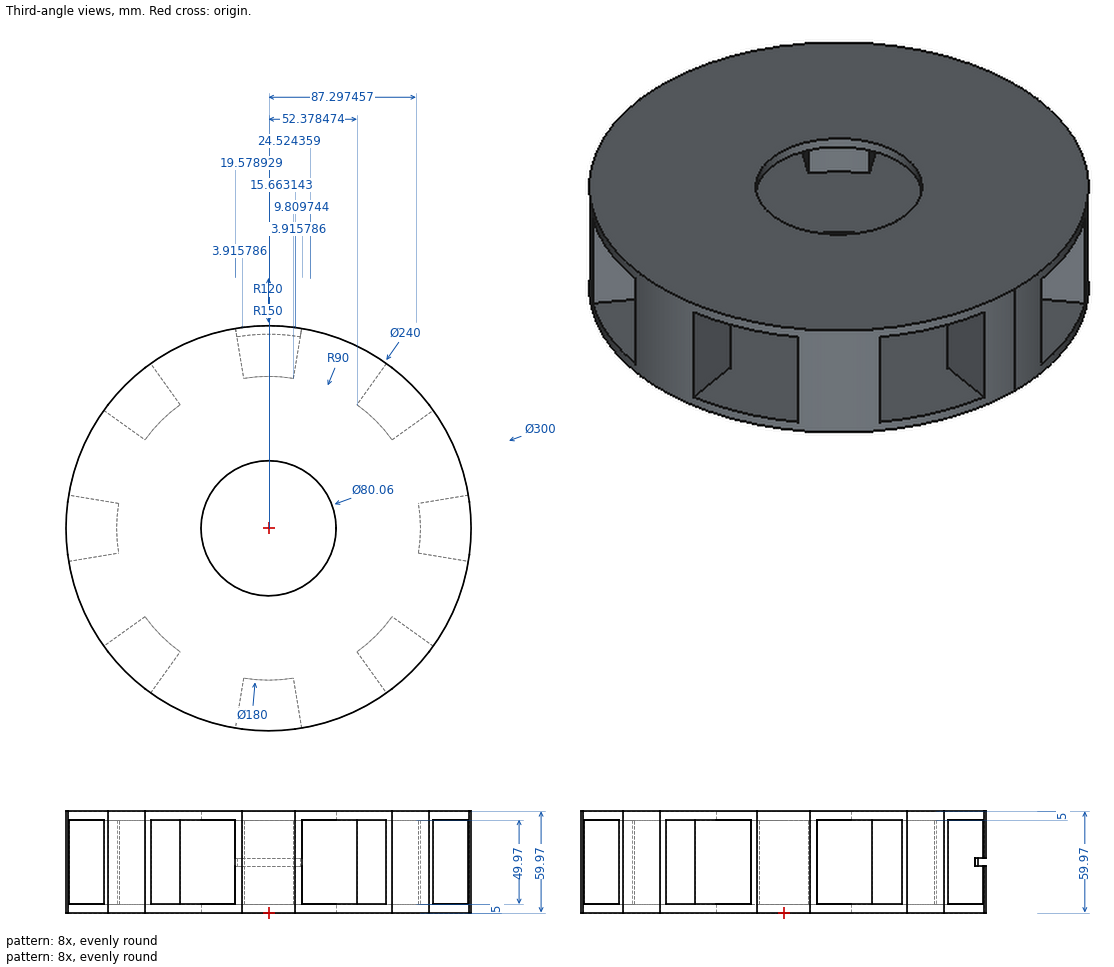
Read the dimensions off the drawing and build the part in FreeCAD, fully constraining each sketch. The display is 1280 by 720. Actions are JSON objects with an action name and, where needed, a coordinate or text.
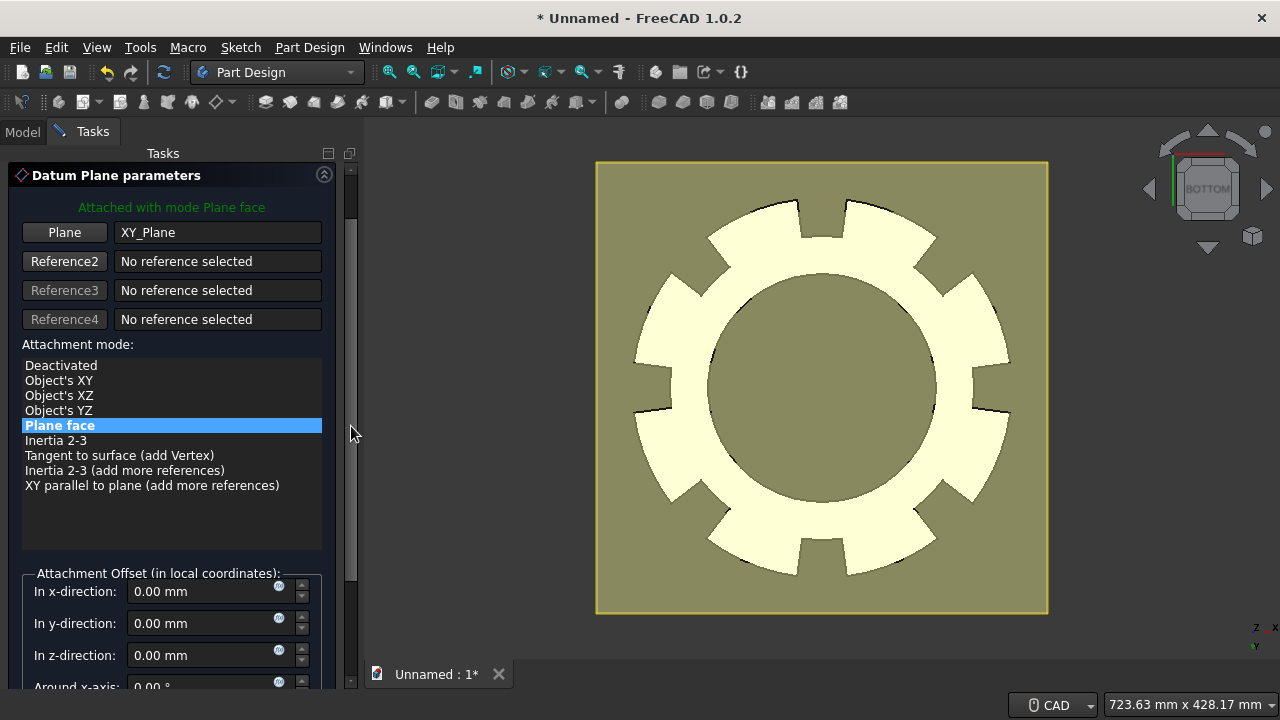
{"action": "triple_click", "coordinate": [210, 595]}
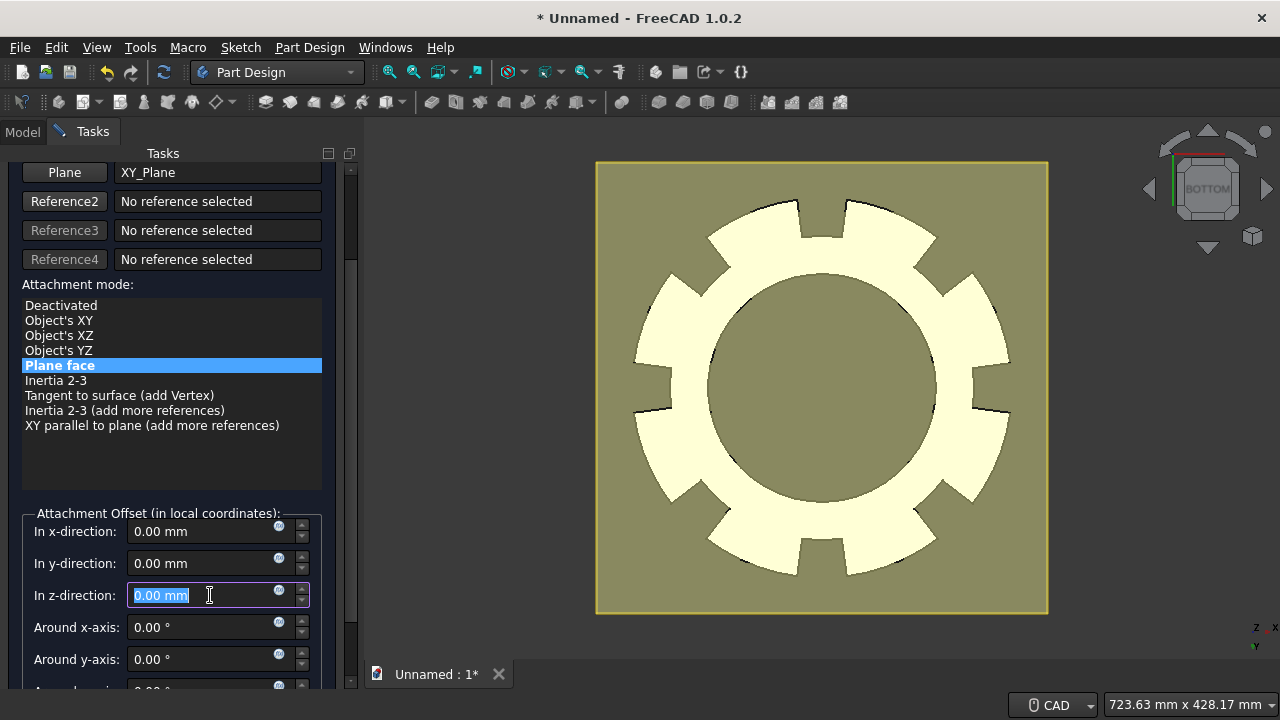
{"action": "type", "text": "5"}
{"action": "key", "text": "Tab"}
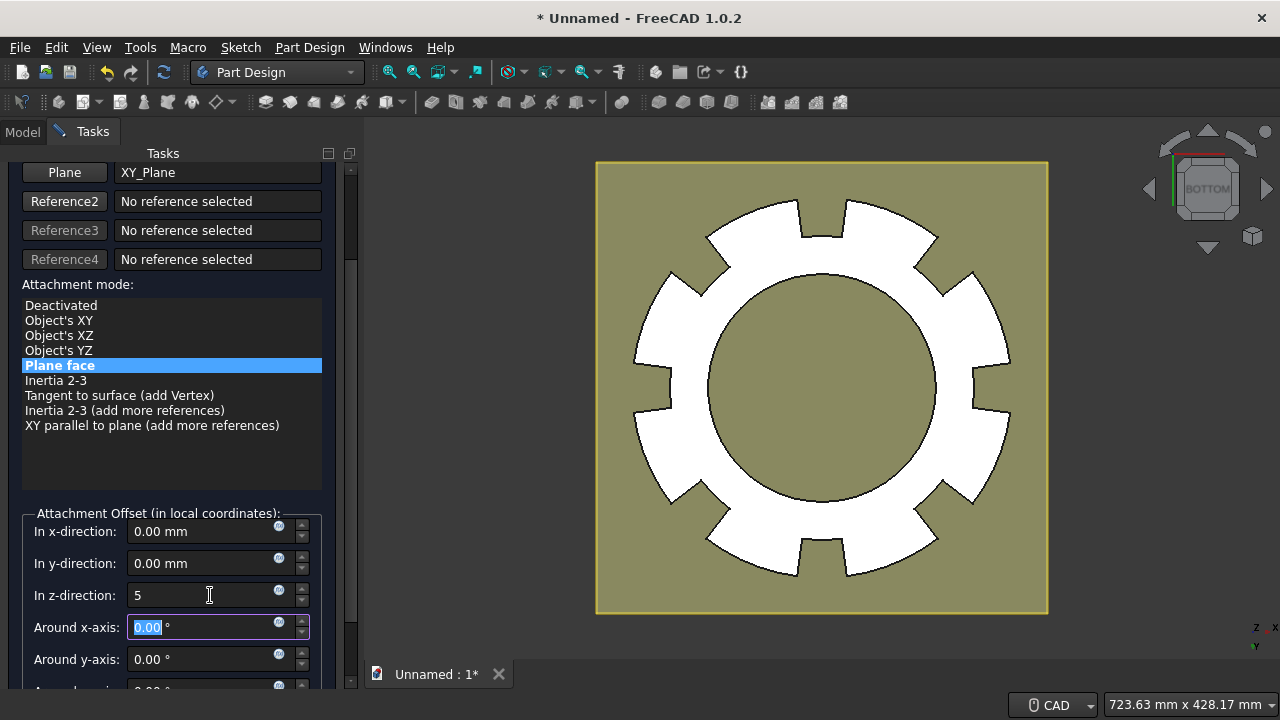
{"action": "scroll", "coordinate": [351, 426], "scroll_direction": "up", "scroll_amount": 3}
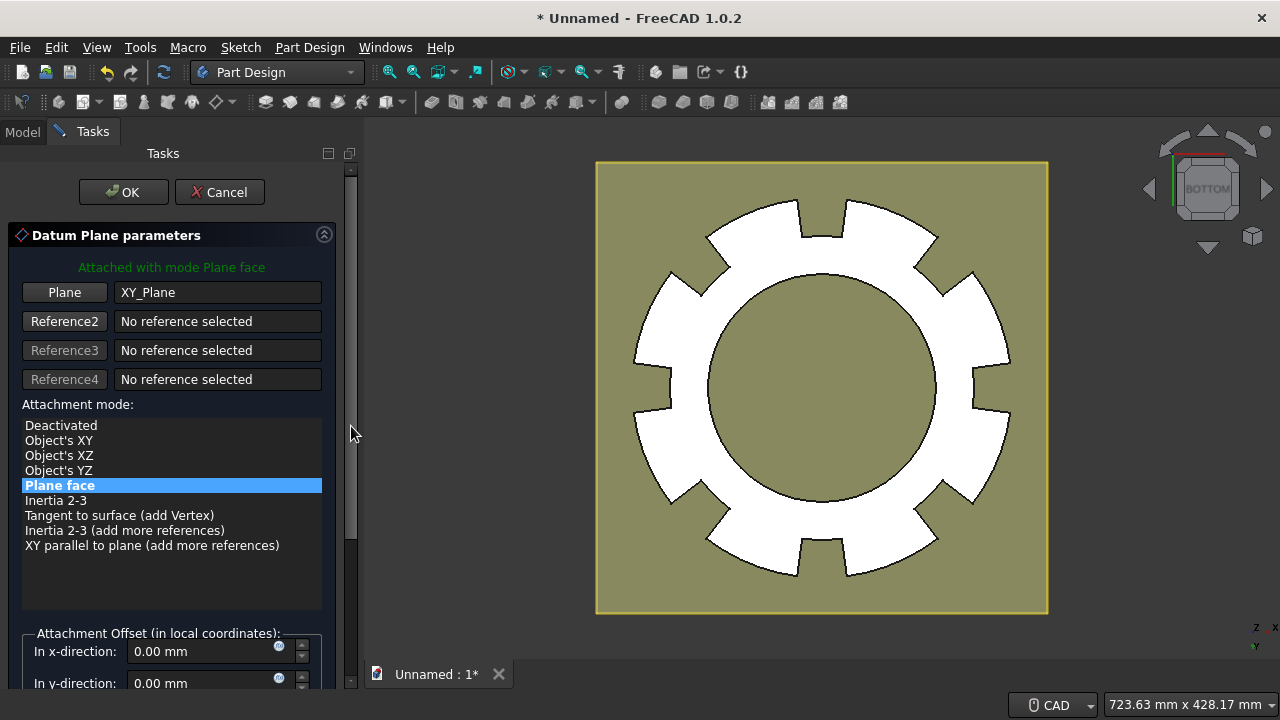
{"action": "left_click", "coordinate": [124, 192]}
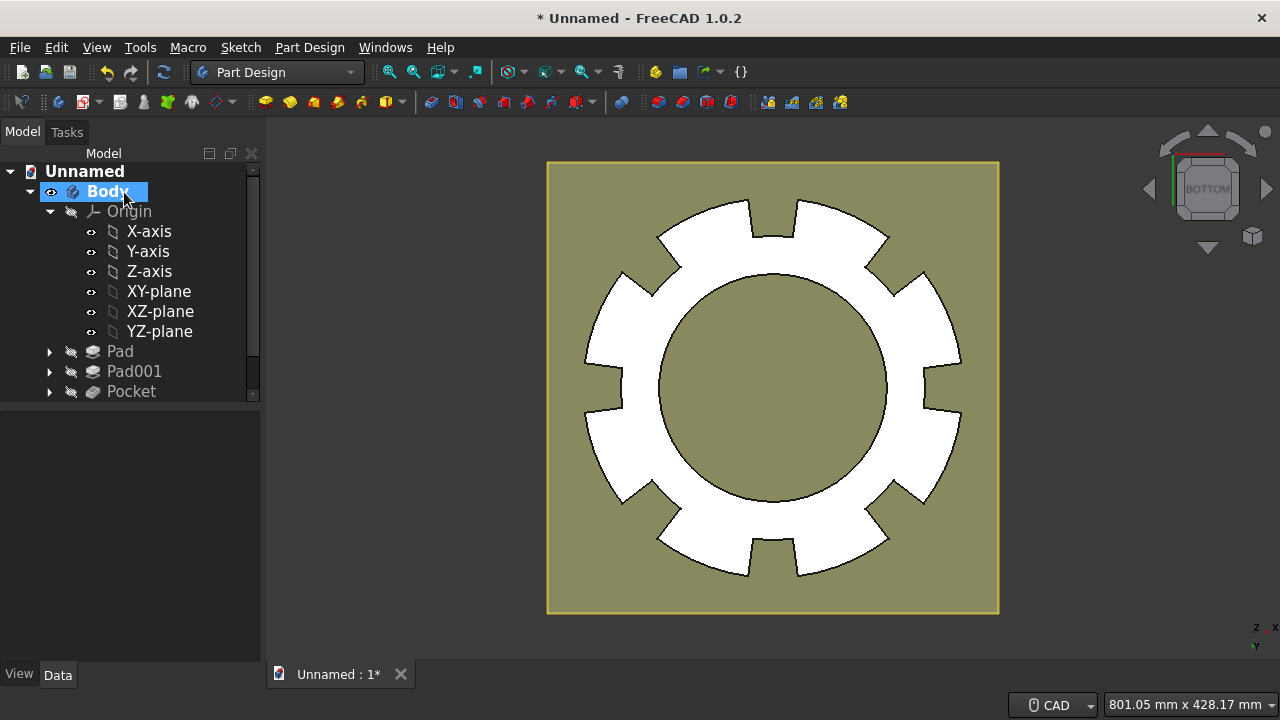
{"action": "scroll", "coordinate": [100, 287], "scroll_direction": "down", "scroll_amount": 3}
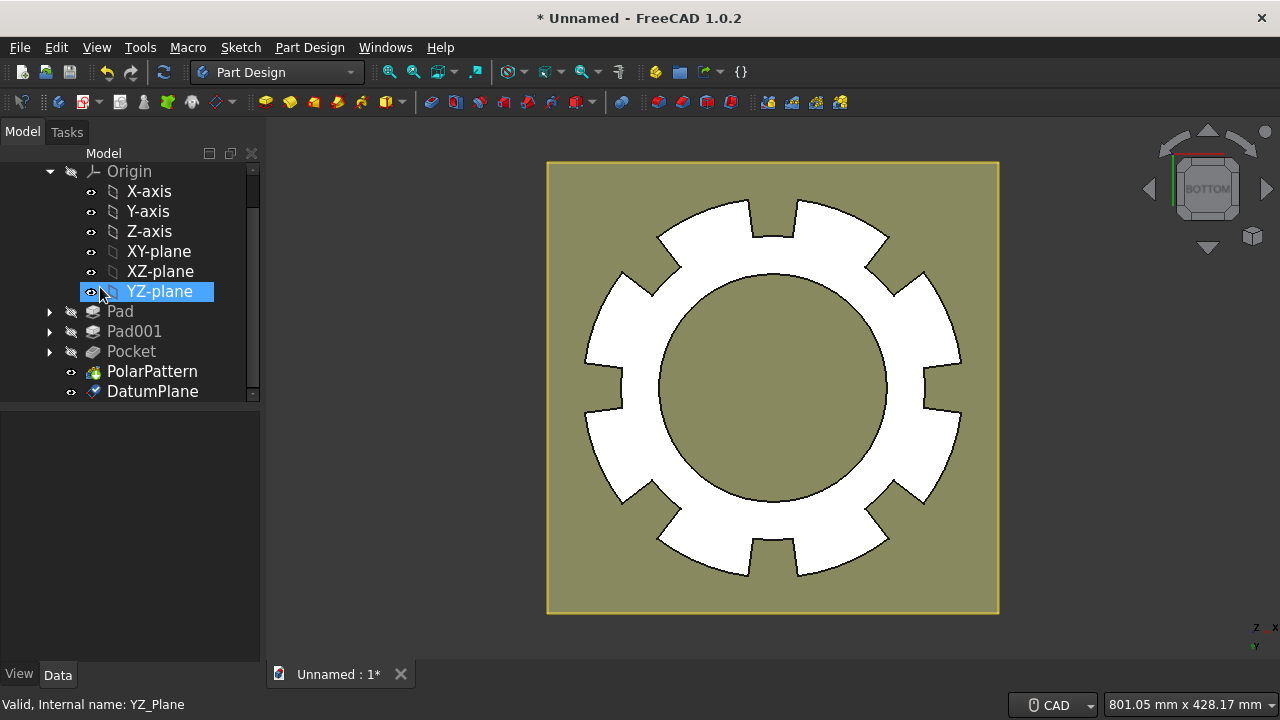
{"action": "left_click", "coordinate": [116, 392]}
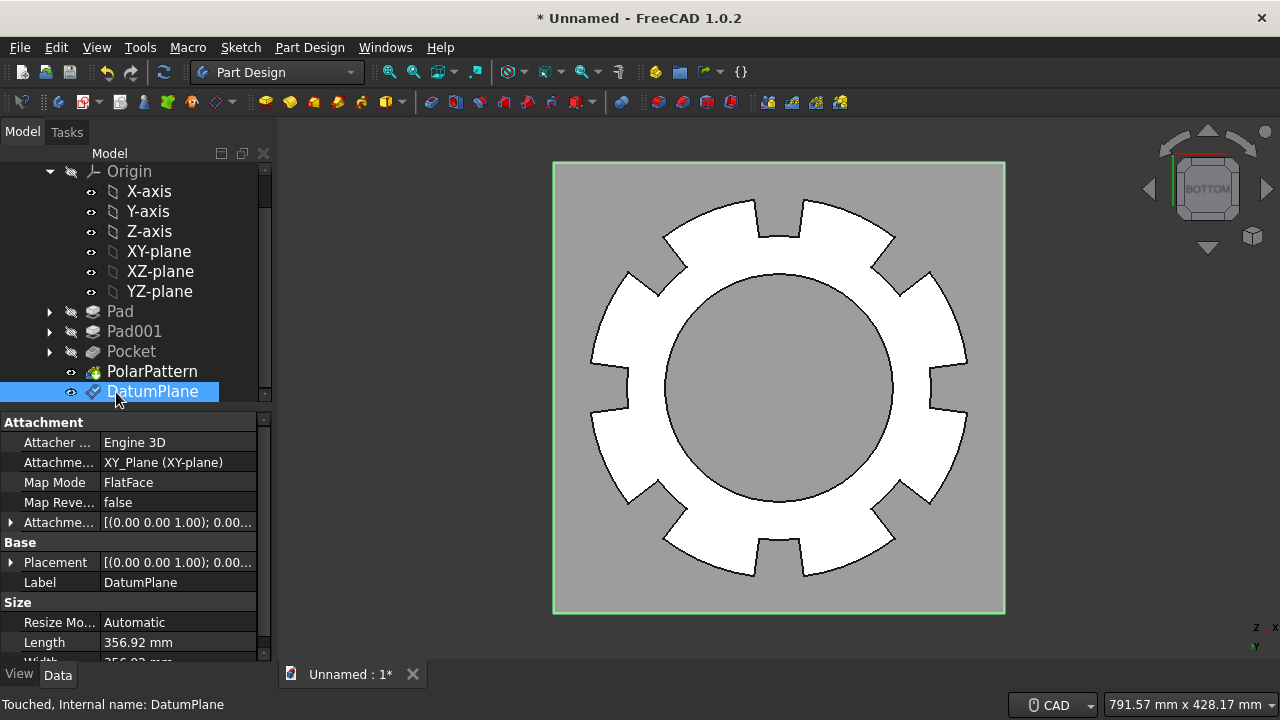
{"action": "left_click", "coordinate": [84, 102]}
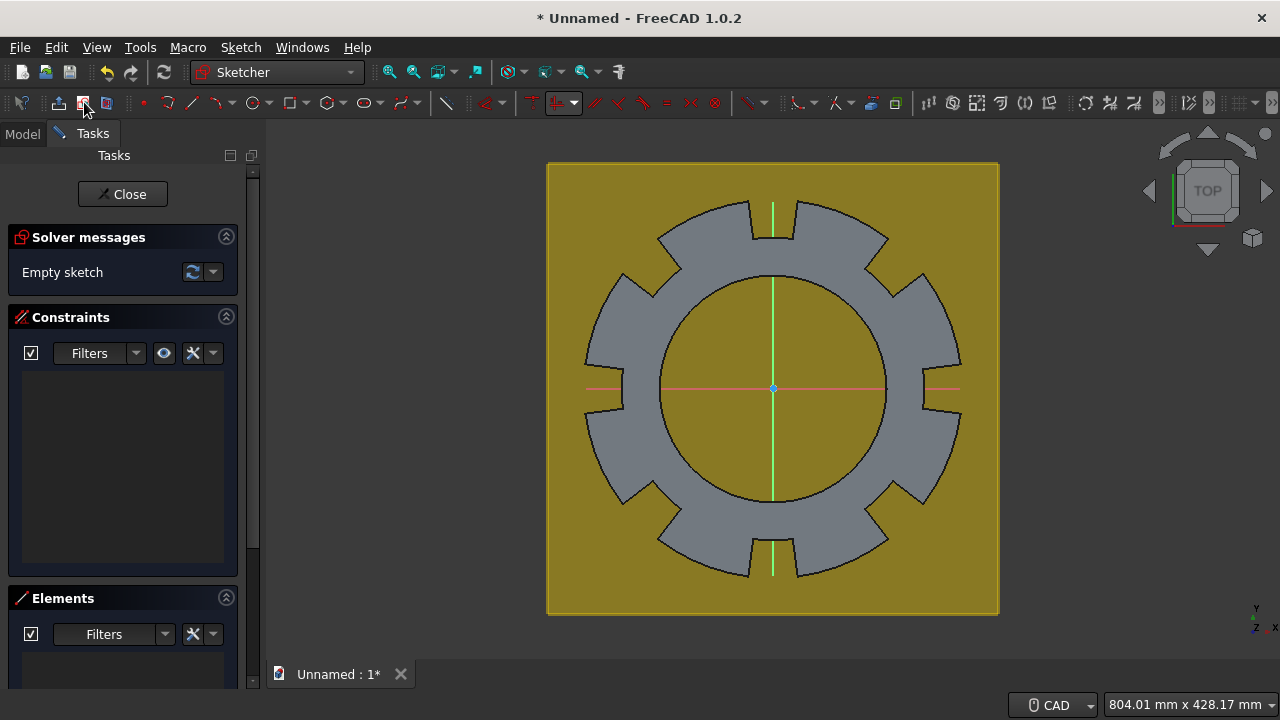
{"action": "left_click", "coordinate": [108, 104]}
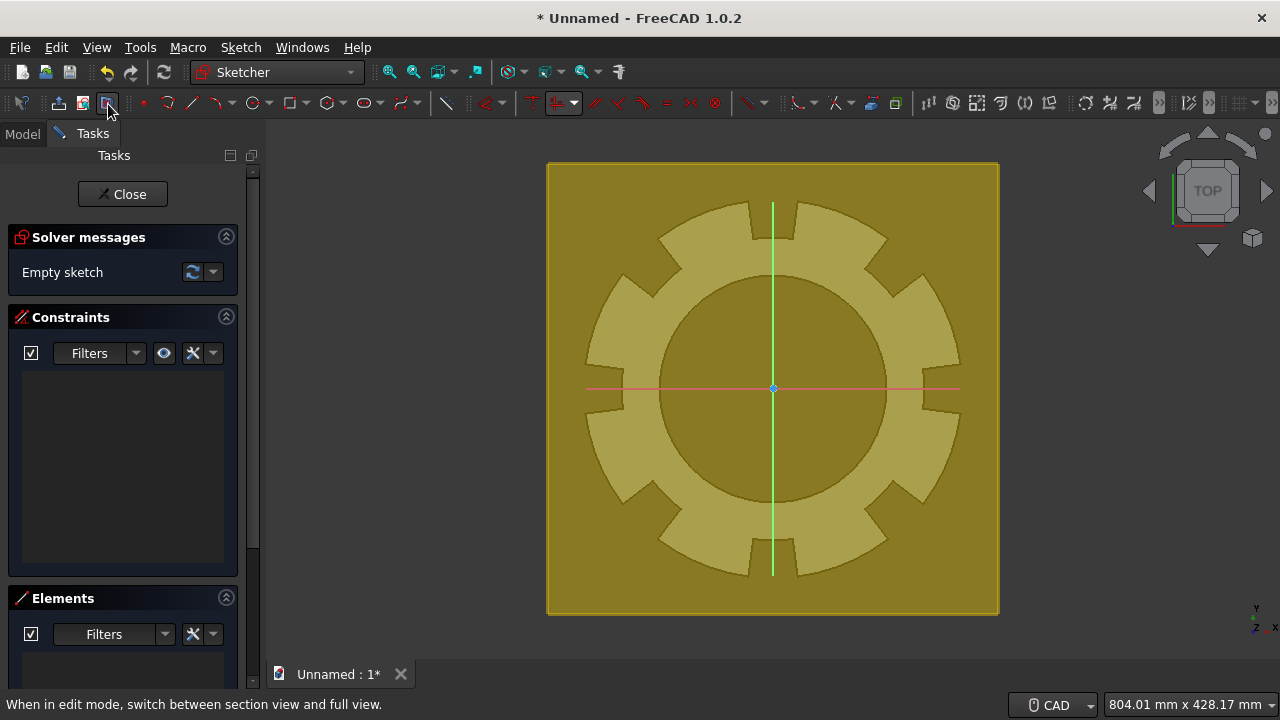
{"action": "scroll", "coordinate": [978, 182], "scroll_direction": "up", "scroll_amount": 3}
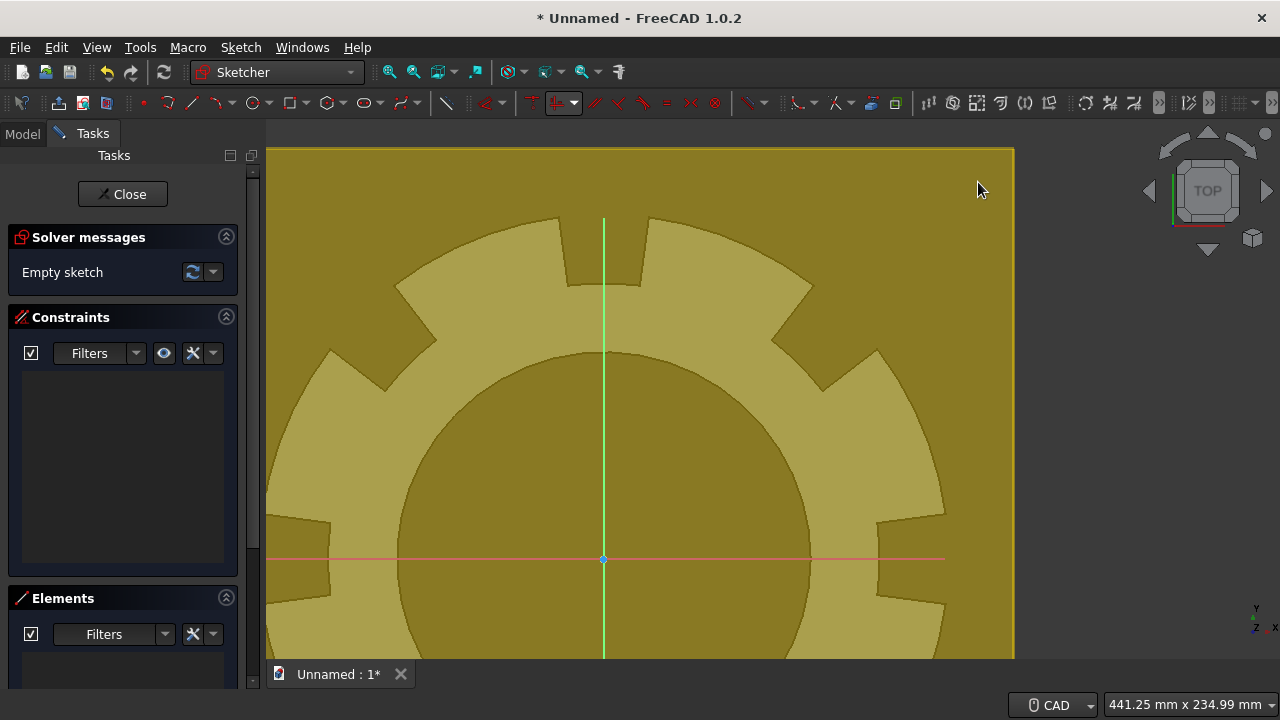
{"action": "left_click", "coordinate": [192, 104]}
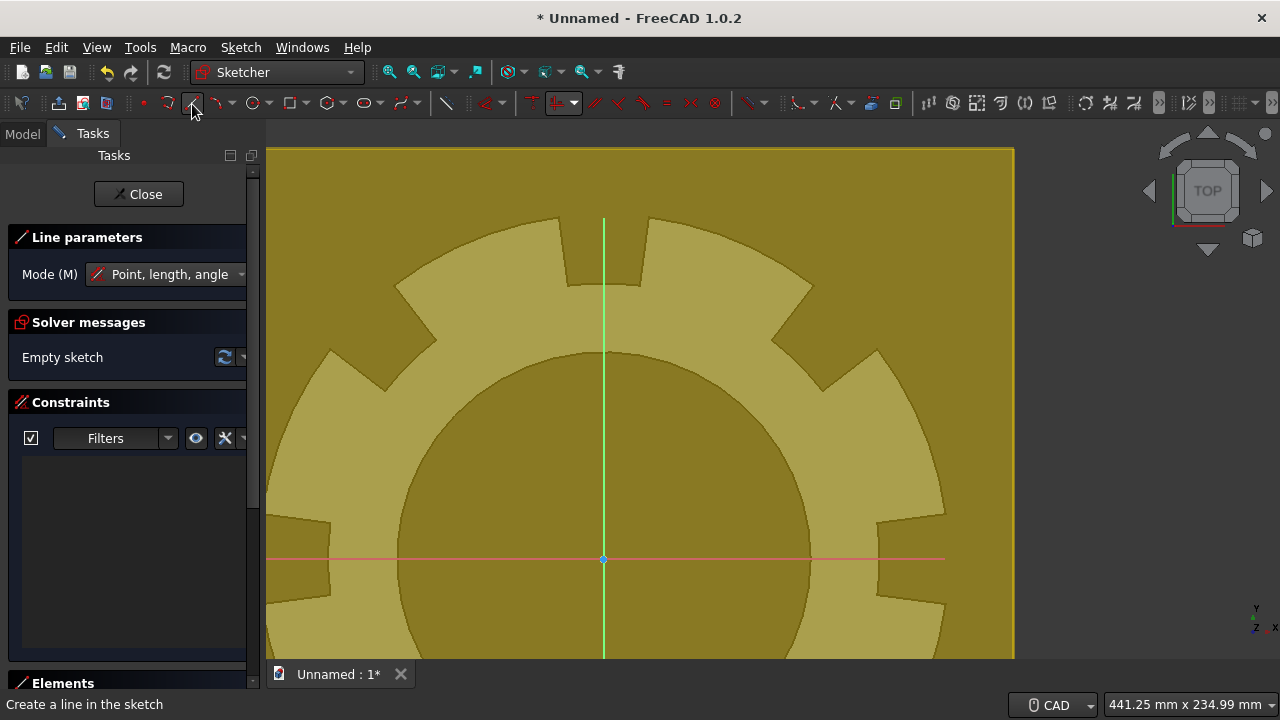
{"action": "left_click", "coordinate": [660, 219]}
{"action": "left_click", "coordinate": [638, 355]}